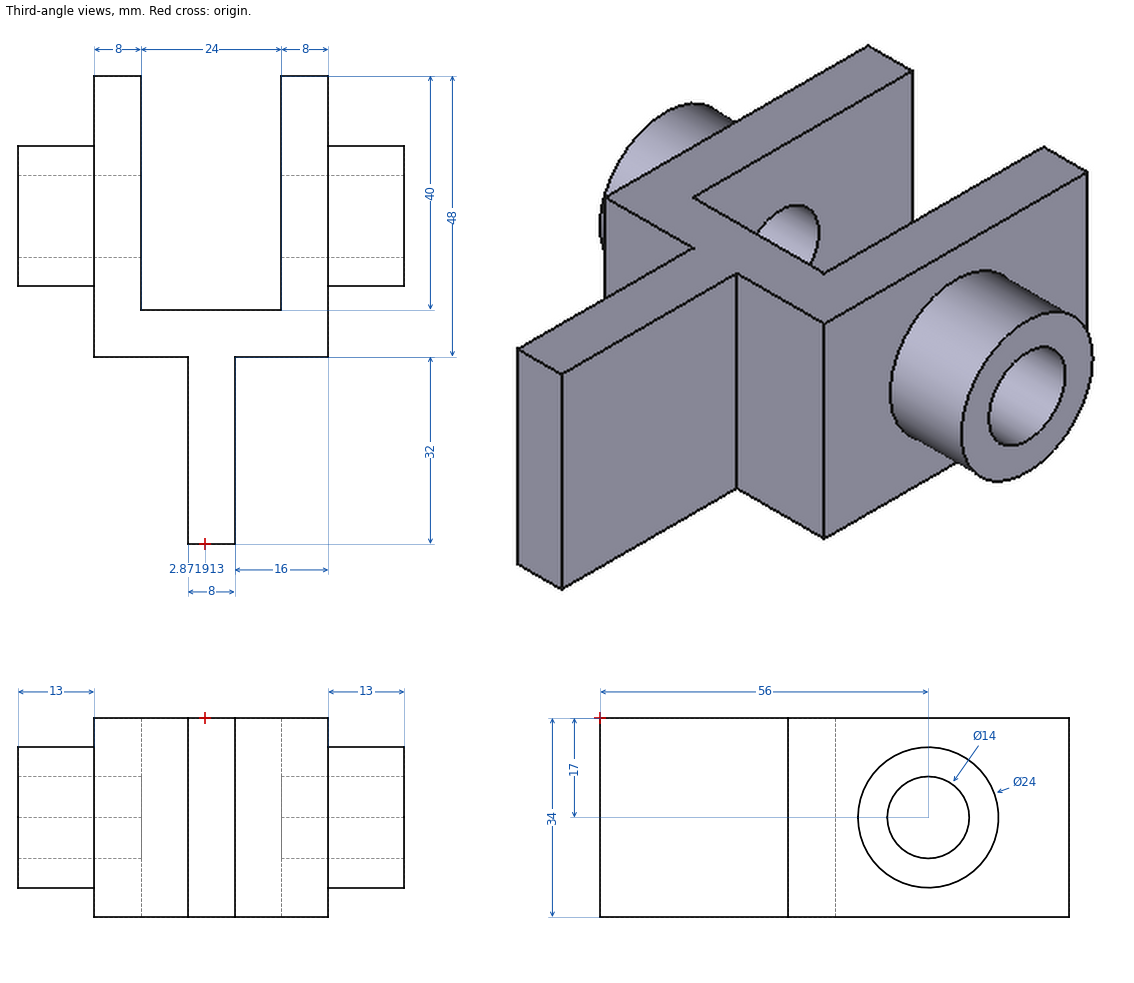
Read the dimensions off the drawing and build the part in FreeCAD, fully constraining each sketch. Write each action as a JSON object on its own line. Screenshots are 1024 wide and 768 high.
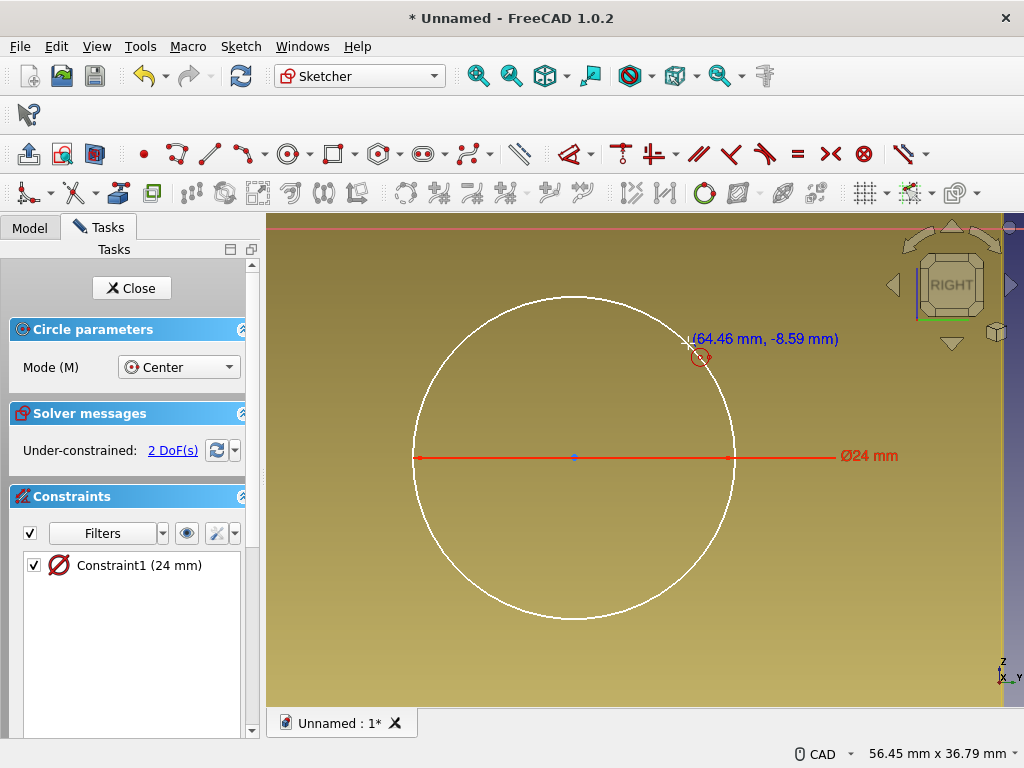
{"action": "left_click", "coordinate": [574, 458]}
{"action": "mouse_move", "coordinate": [641, 390]}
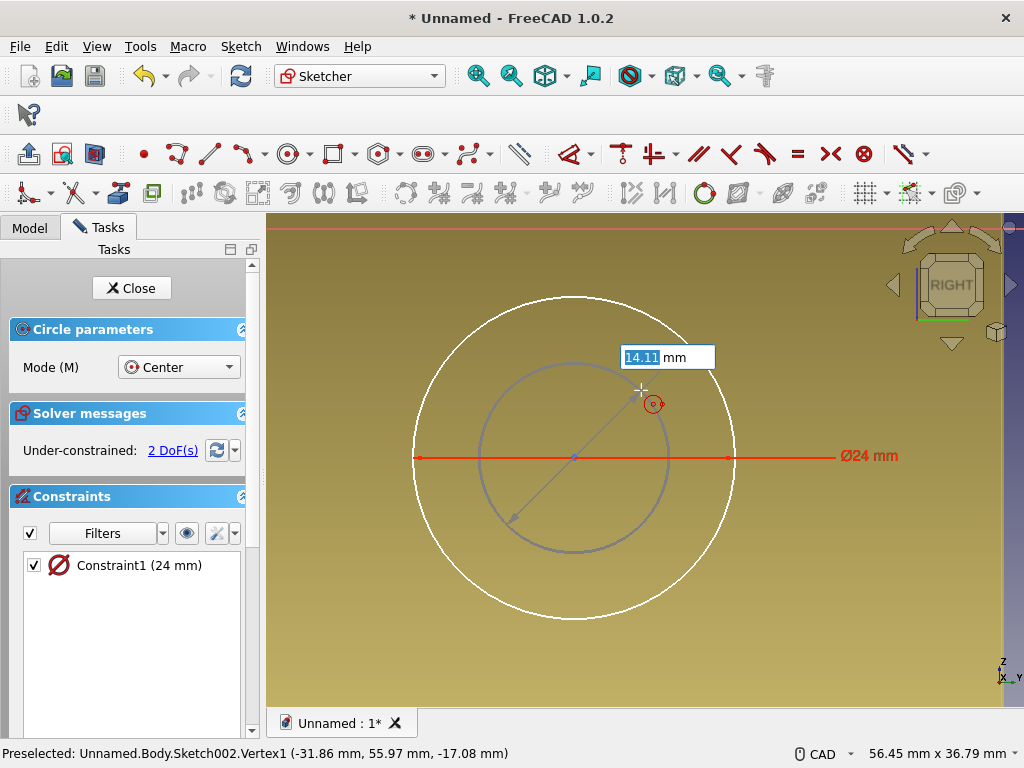
{"action": "type", "text": "14"}
{"action": "key", "text": "Return"}
{"action": "key", "text": "Escape"}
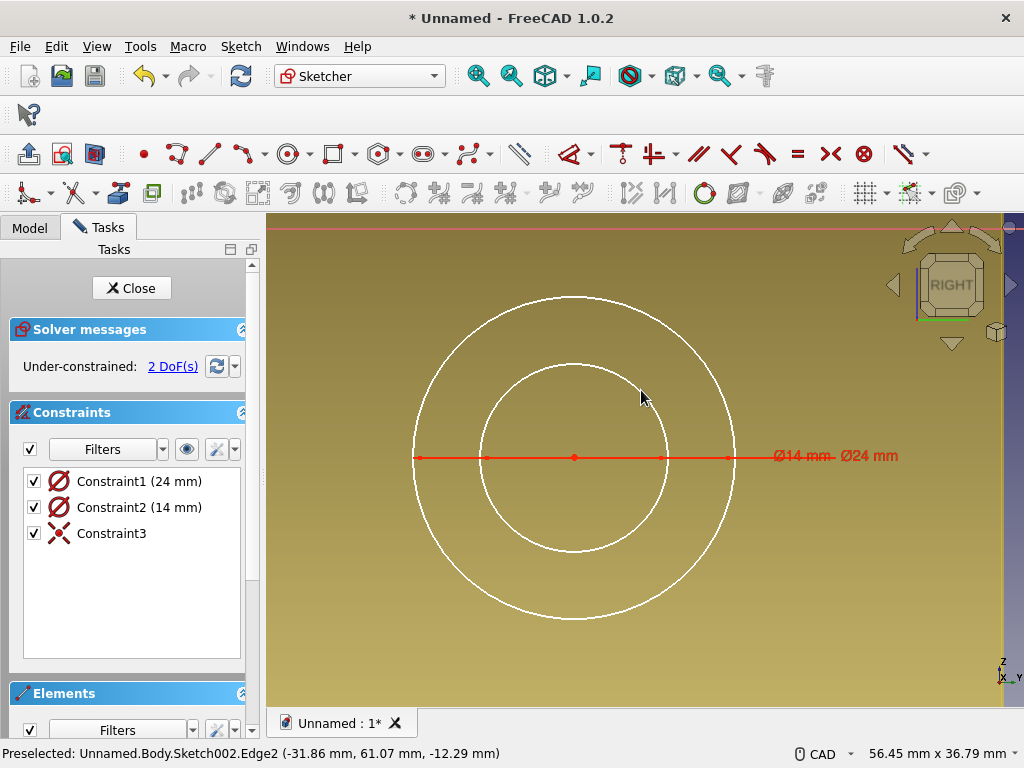
{"action": "left_click", "coordinate": [568, 154]}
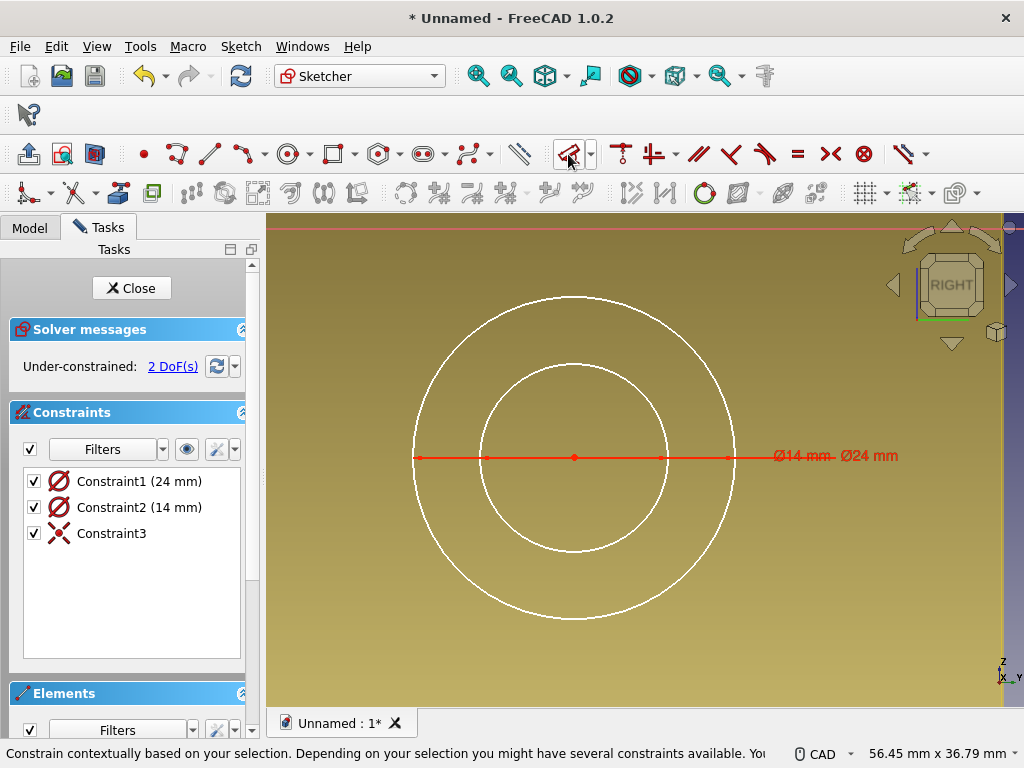
{"action": "left_click", "coordinate": [574, 458]}
{"action": "left_click", "coordinate": [434, 492]}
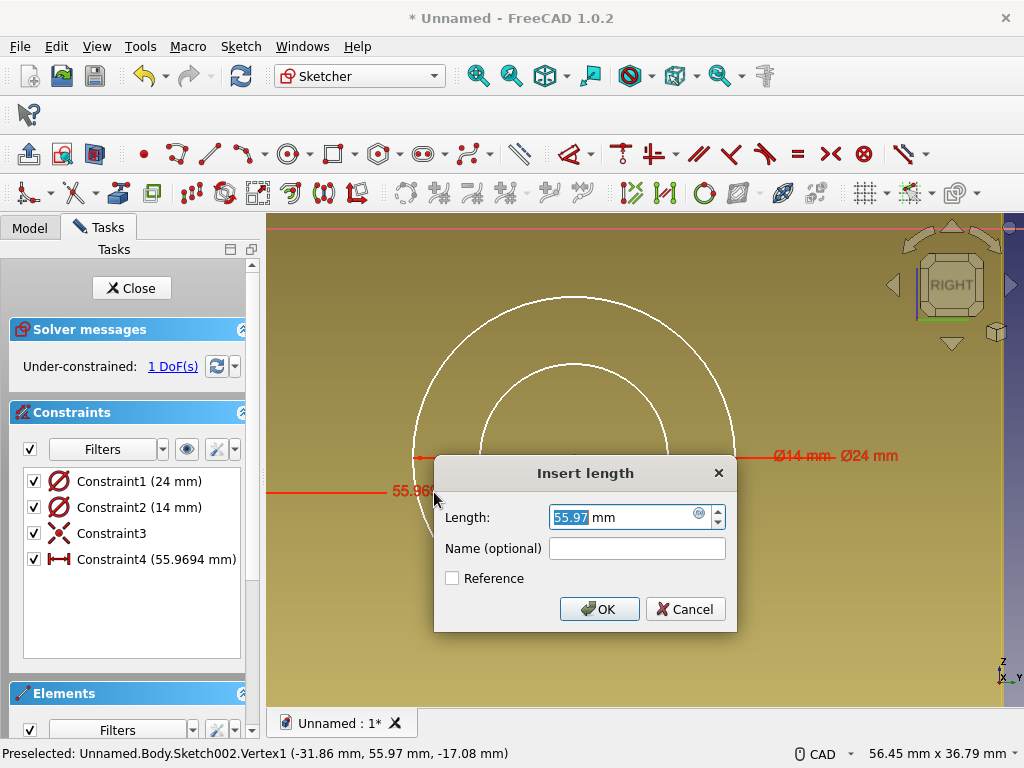
{"action": "type", "text": "56"}
{"action": "key", "text": "Return"}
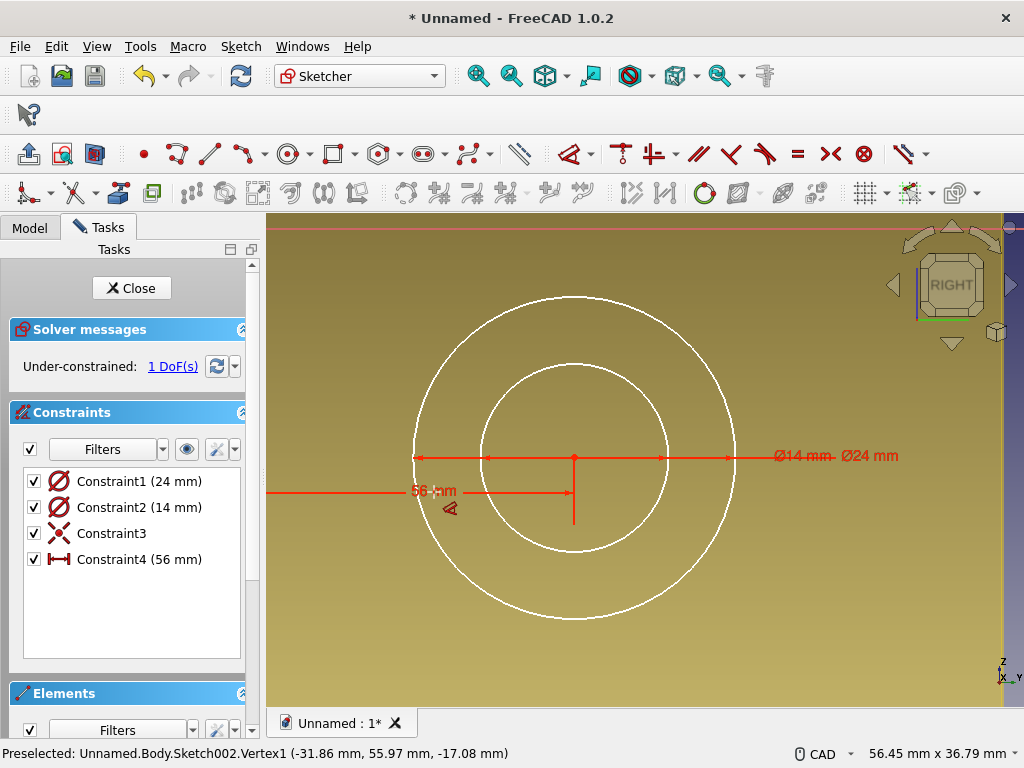
{"action": "left_click", "coordinate": [574, 458]}
{"action": "left_click", "coordinate": [608, 349]}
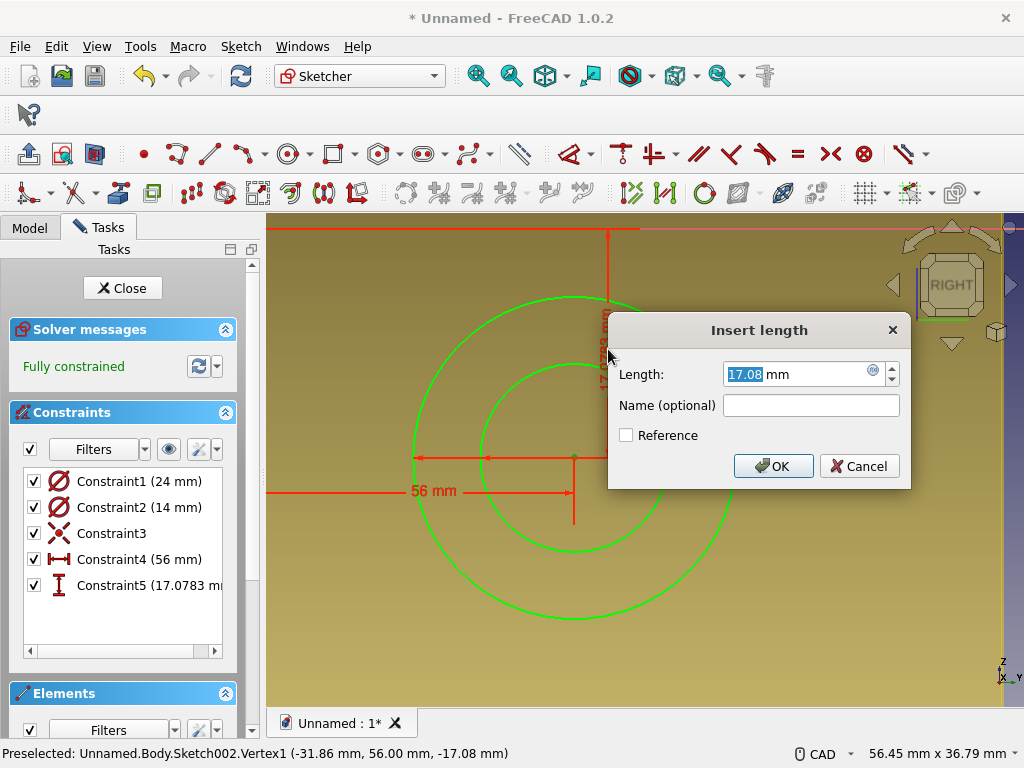
{"action": "type", "text": "17"}
{"action": "key", "text": "Return"}
{"action": "key", "text": "Escape"}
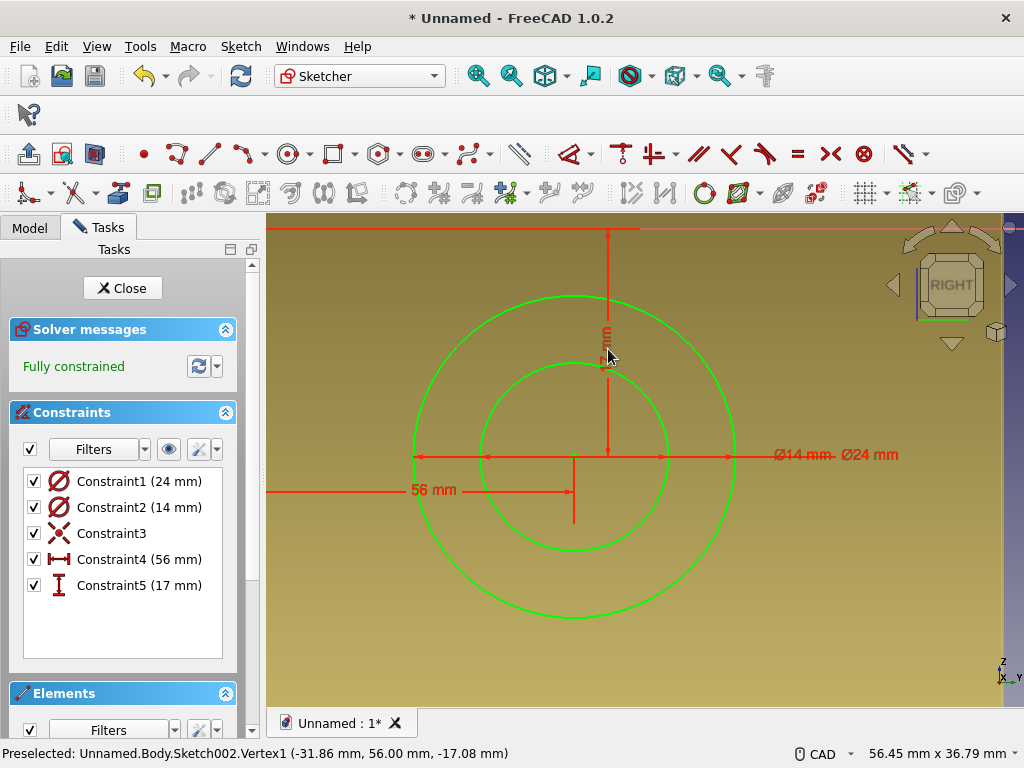
{"action": "left_click", "coordinate": [123, 288]}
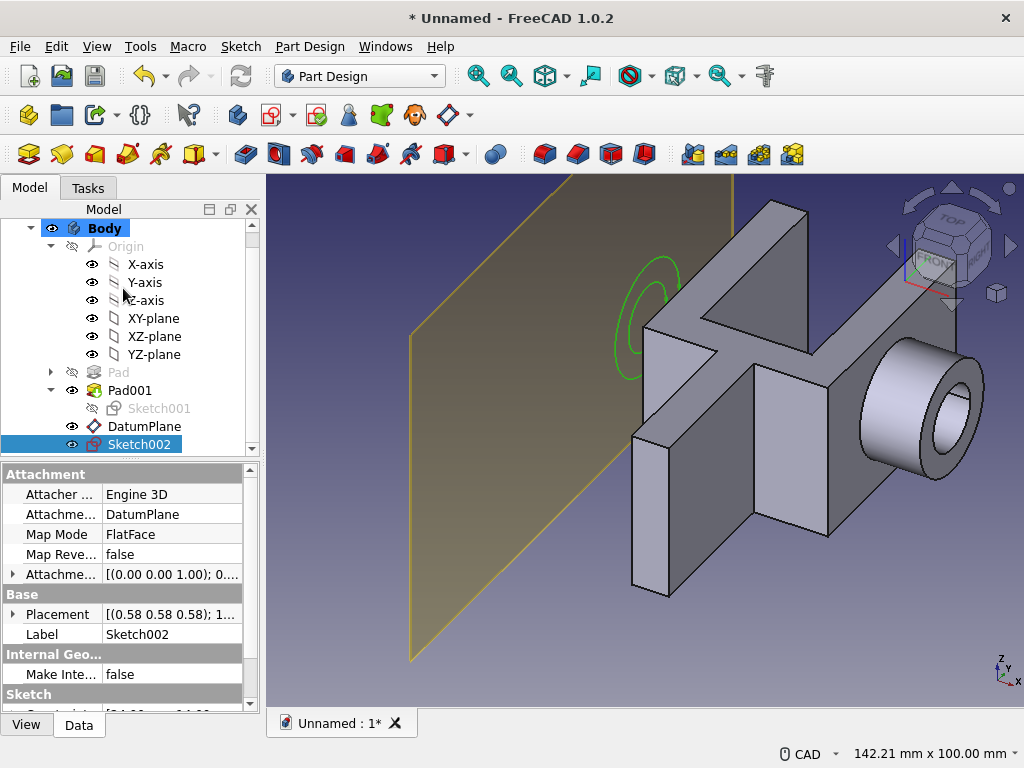
{"action": "left_click", "coordinate": [29, 154]}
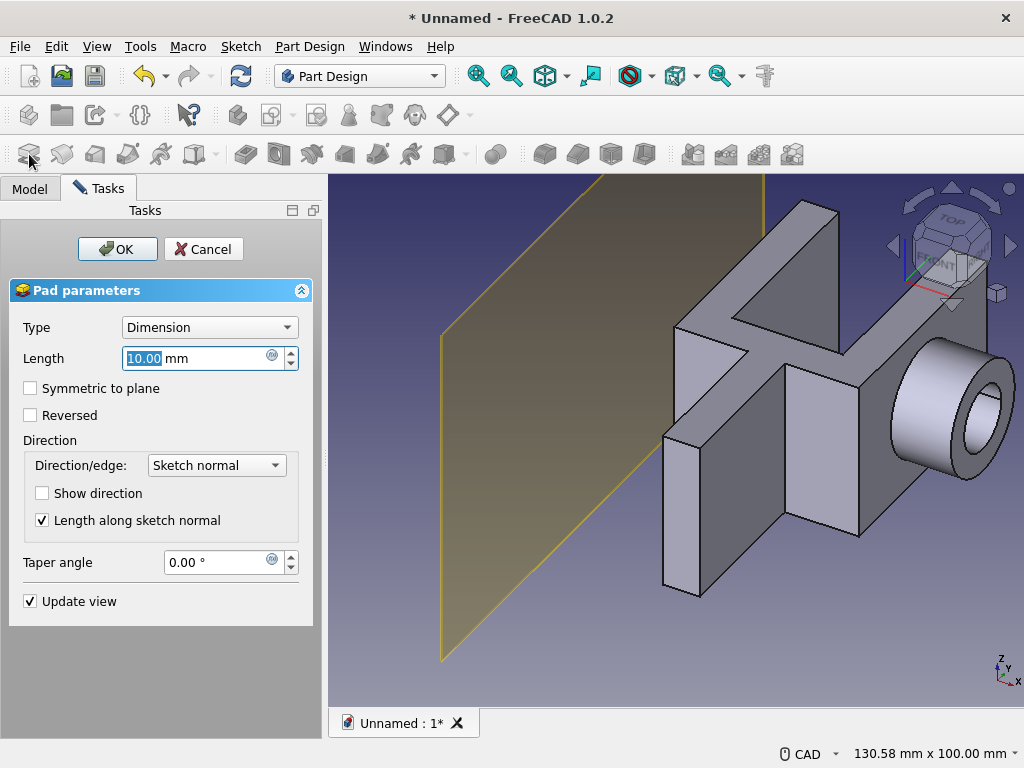
{"action": "type", "text": "13"}
{"action": "key", "text": "Tab"}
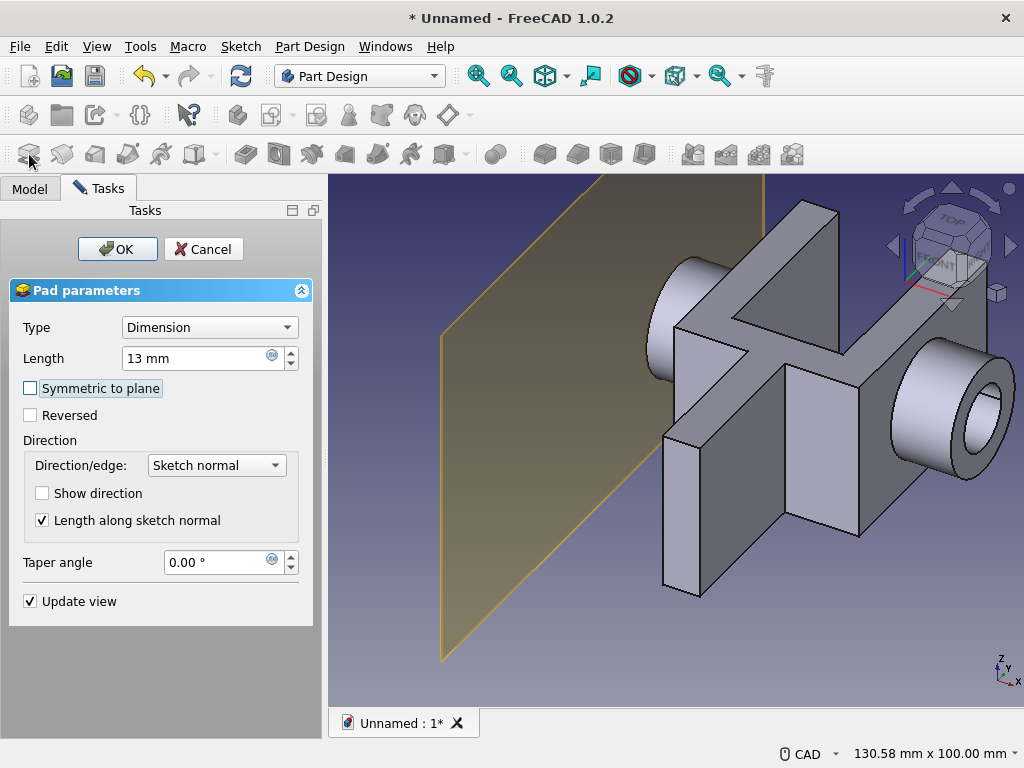
{"action": "left_click", "coordinate": [118, 249]}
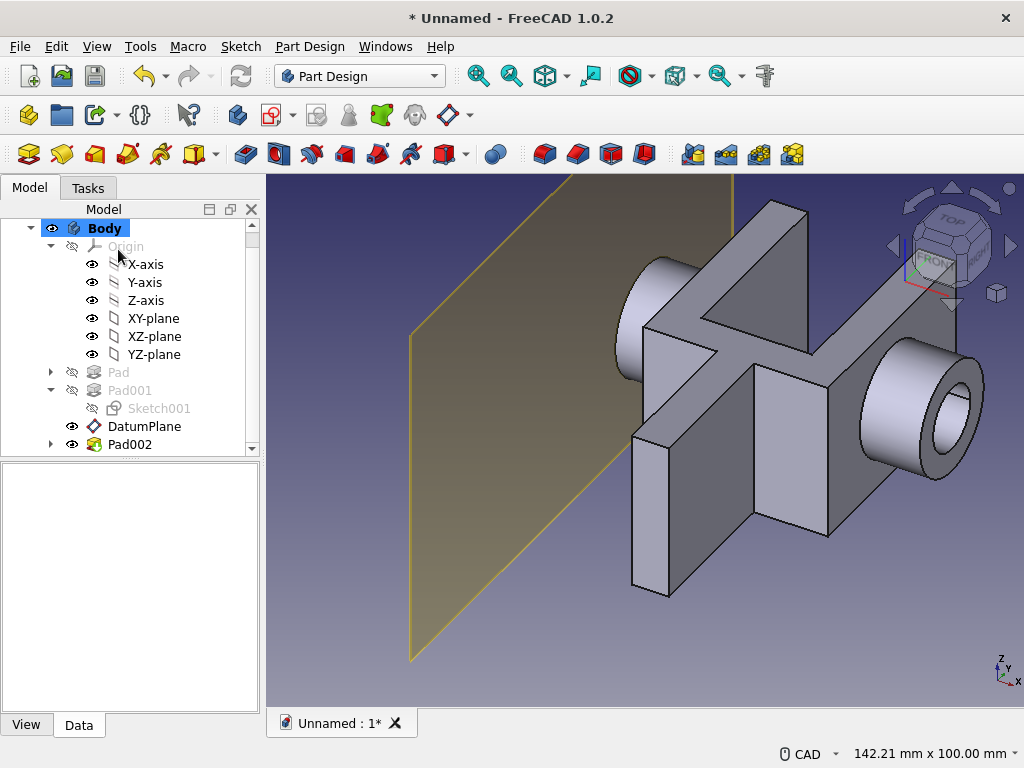
{"action": "left_click", "coordinate": [117, 426]}
{"action": "key", "text": "space"}